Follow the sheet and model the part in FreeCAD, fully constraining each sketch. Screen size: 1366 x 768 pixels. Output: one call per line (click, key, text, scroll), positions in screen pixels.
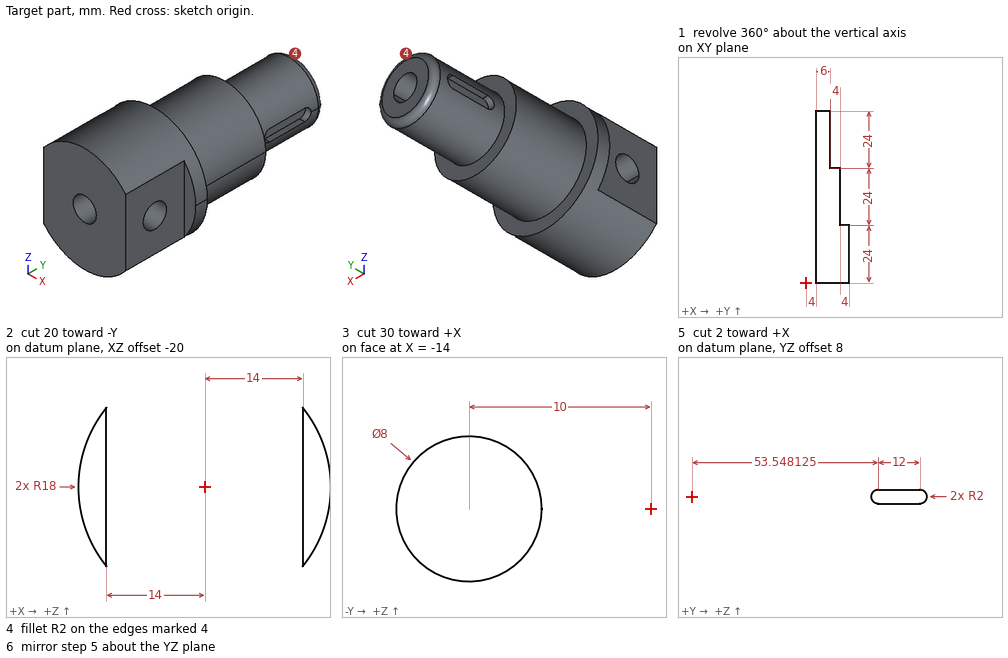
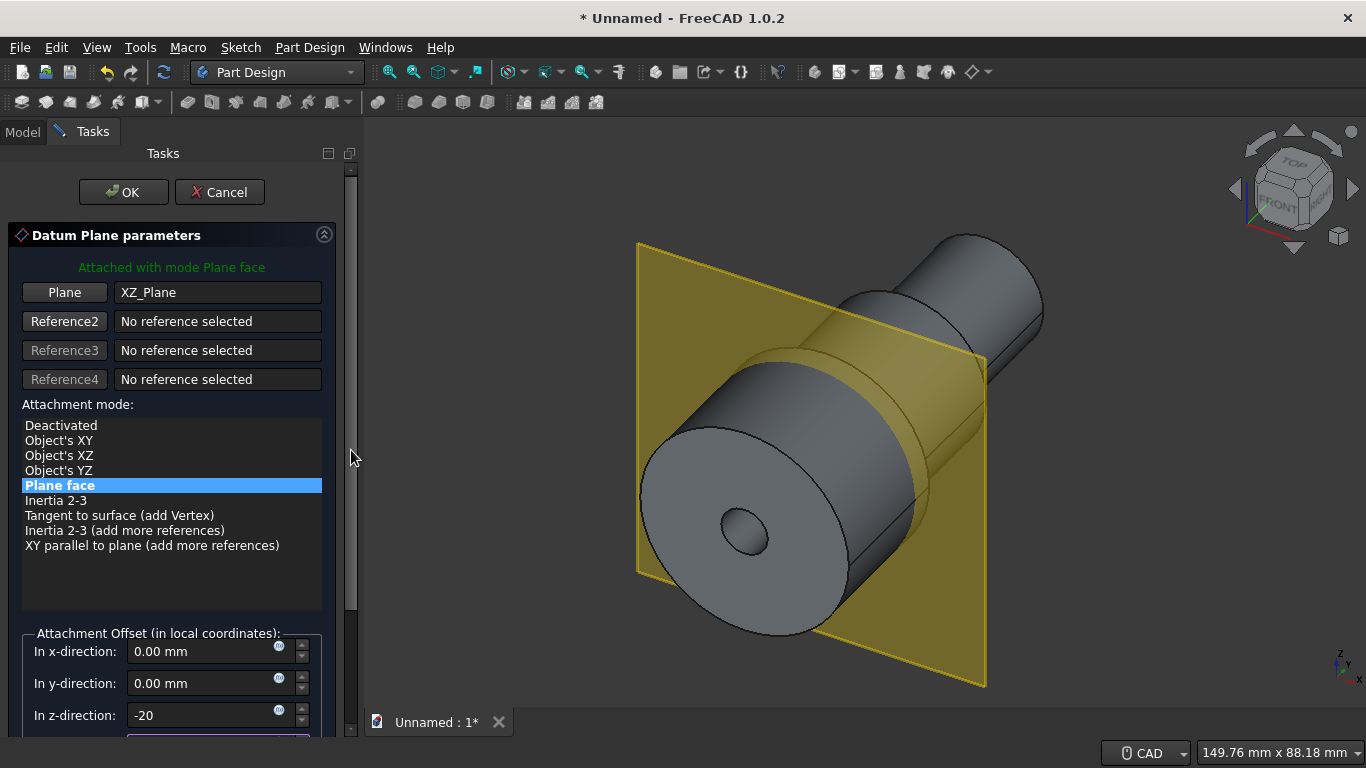
click(124, 192)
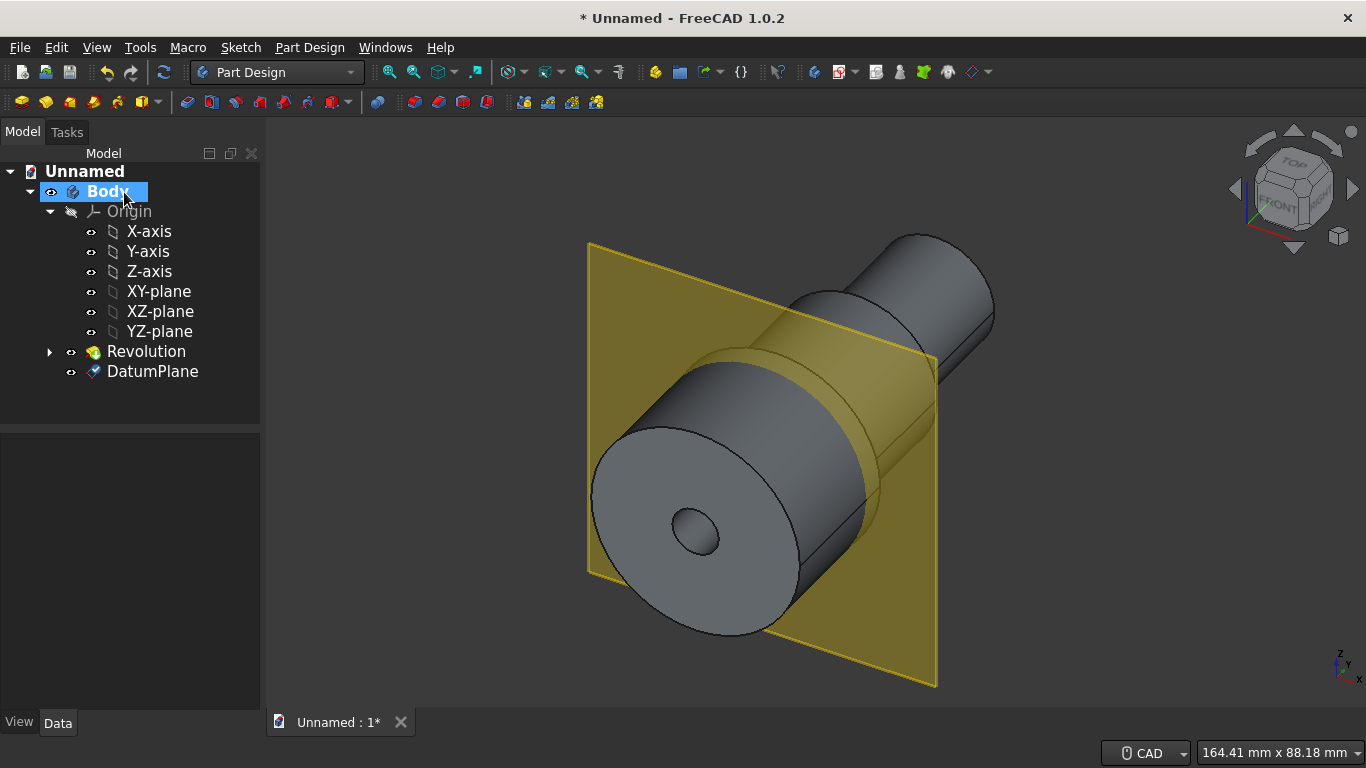
click(116, 372)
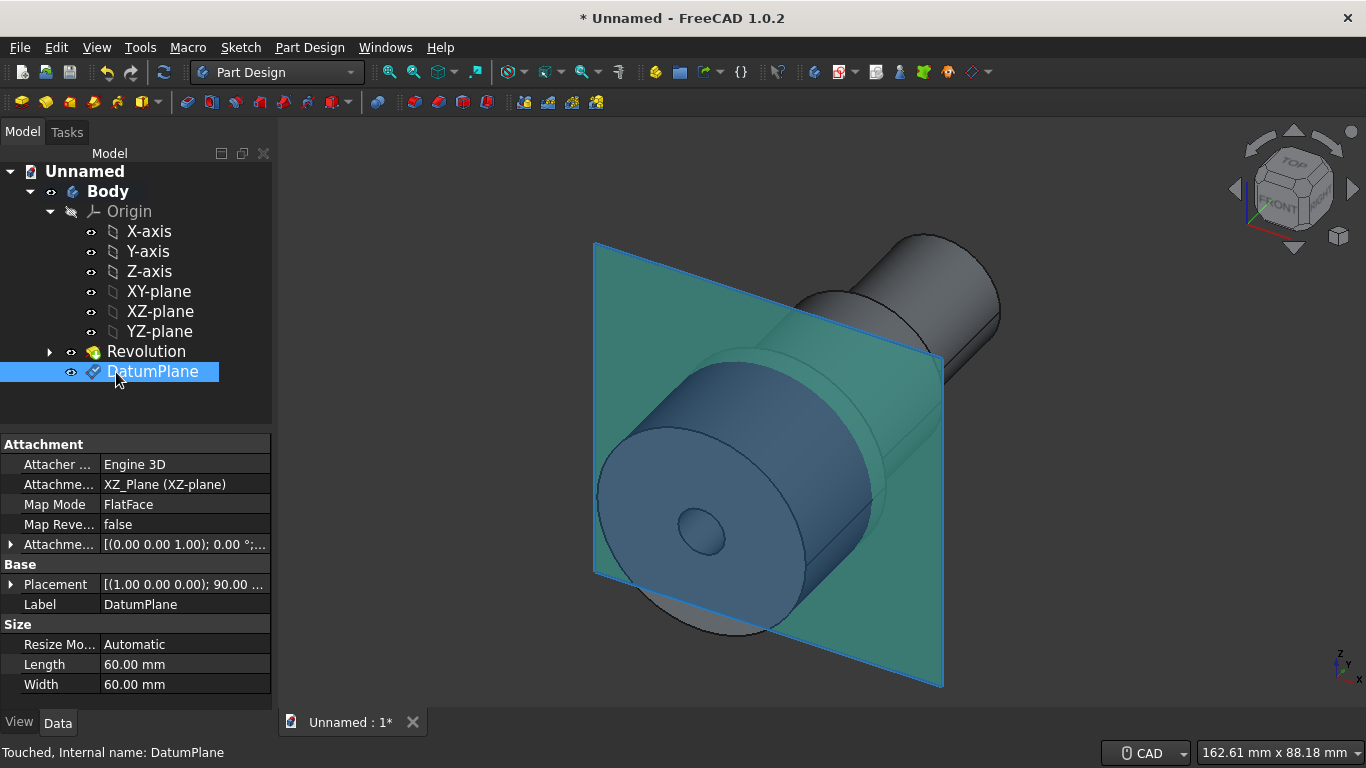
click(840, 72)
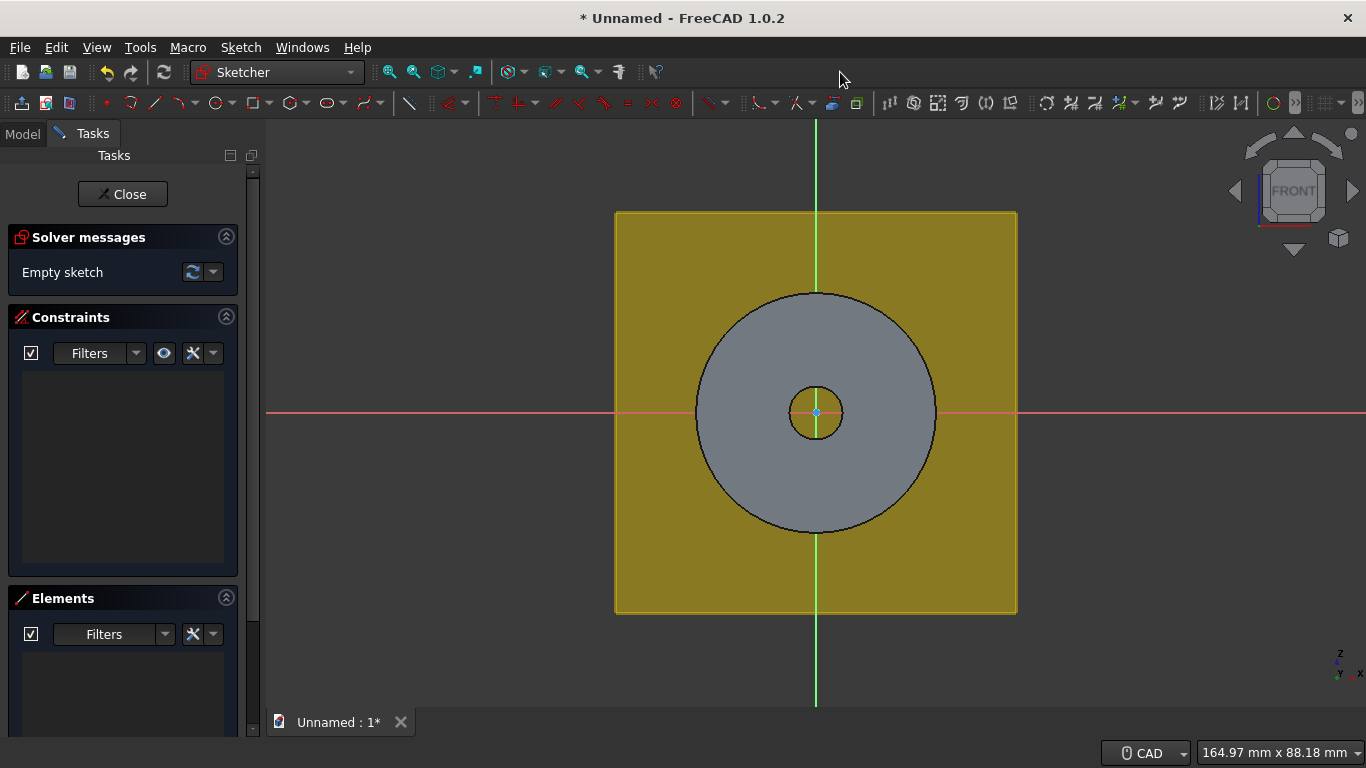
click(70, 104)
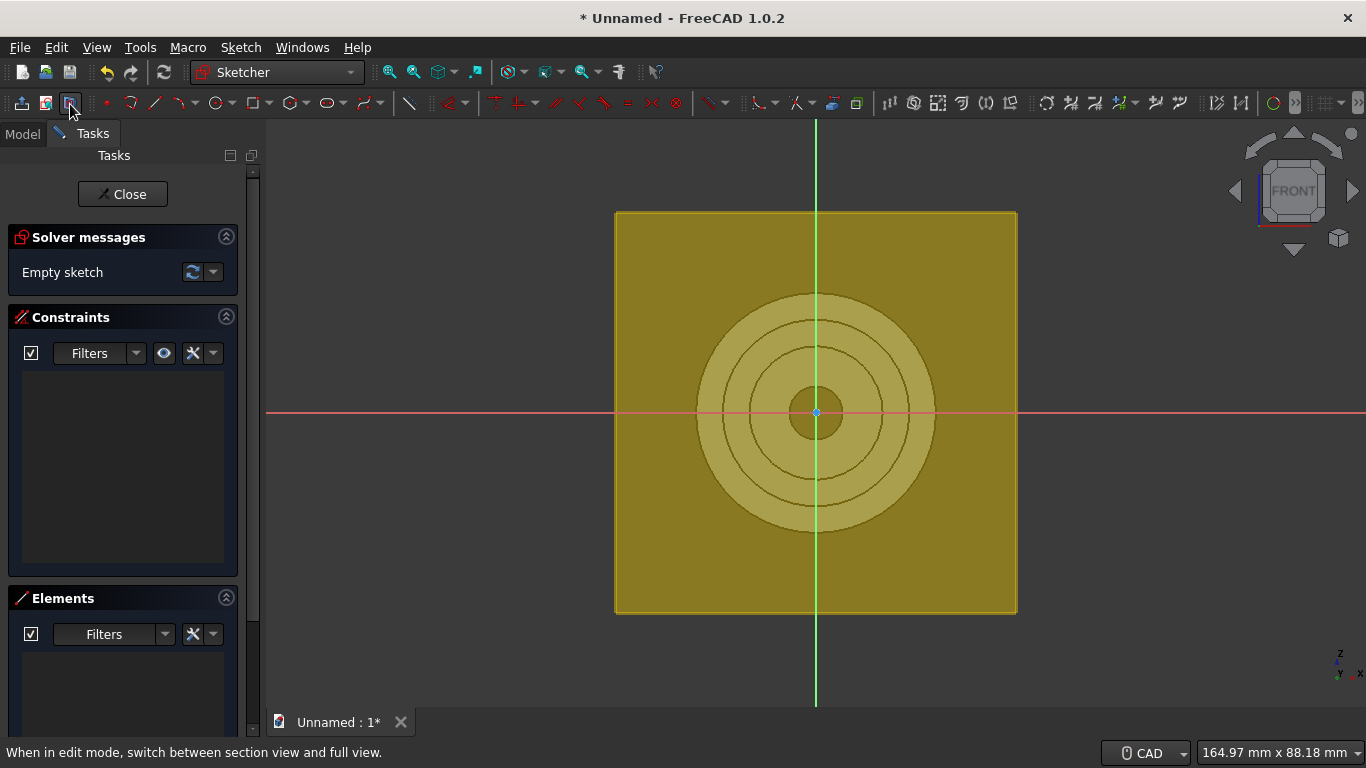
scroll(856, 413, up, 5)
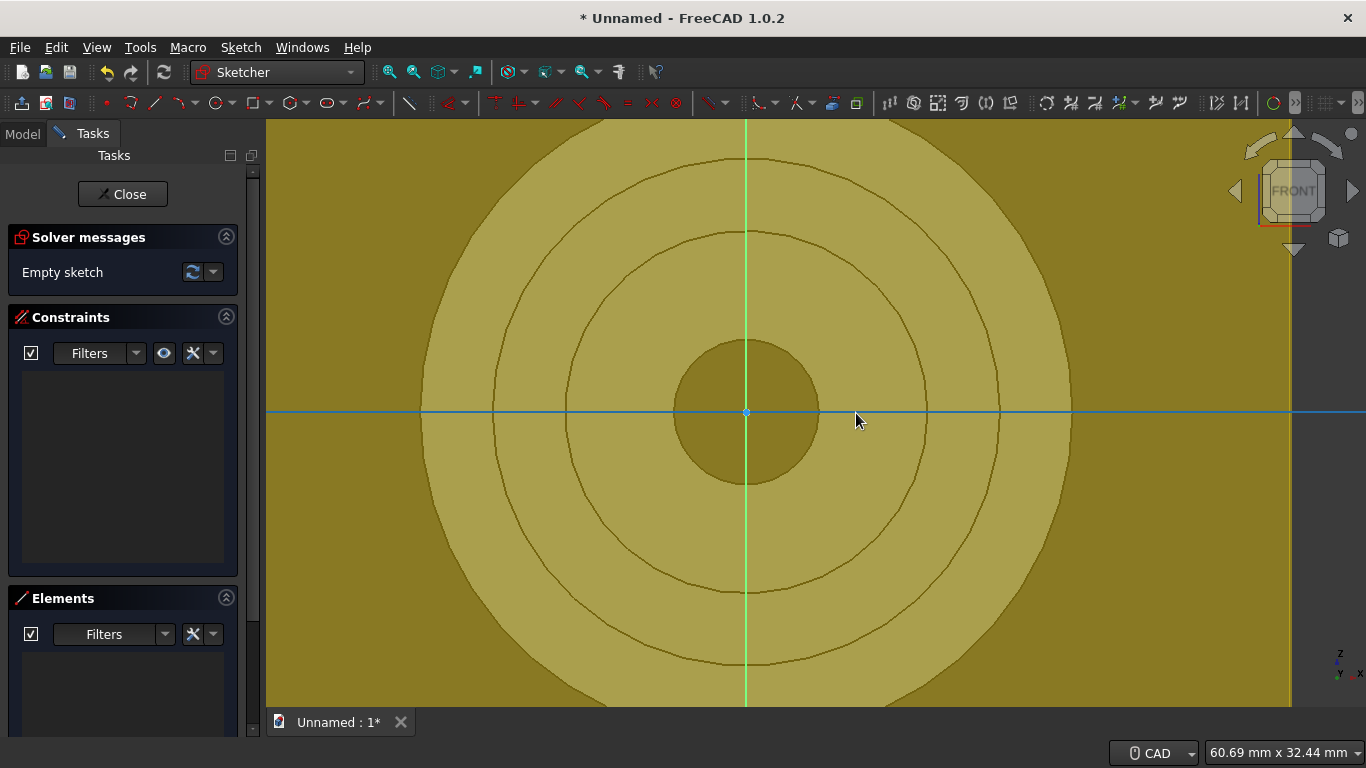
click(156, 104)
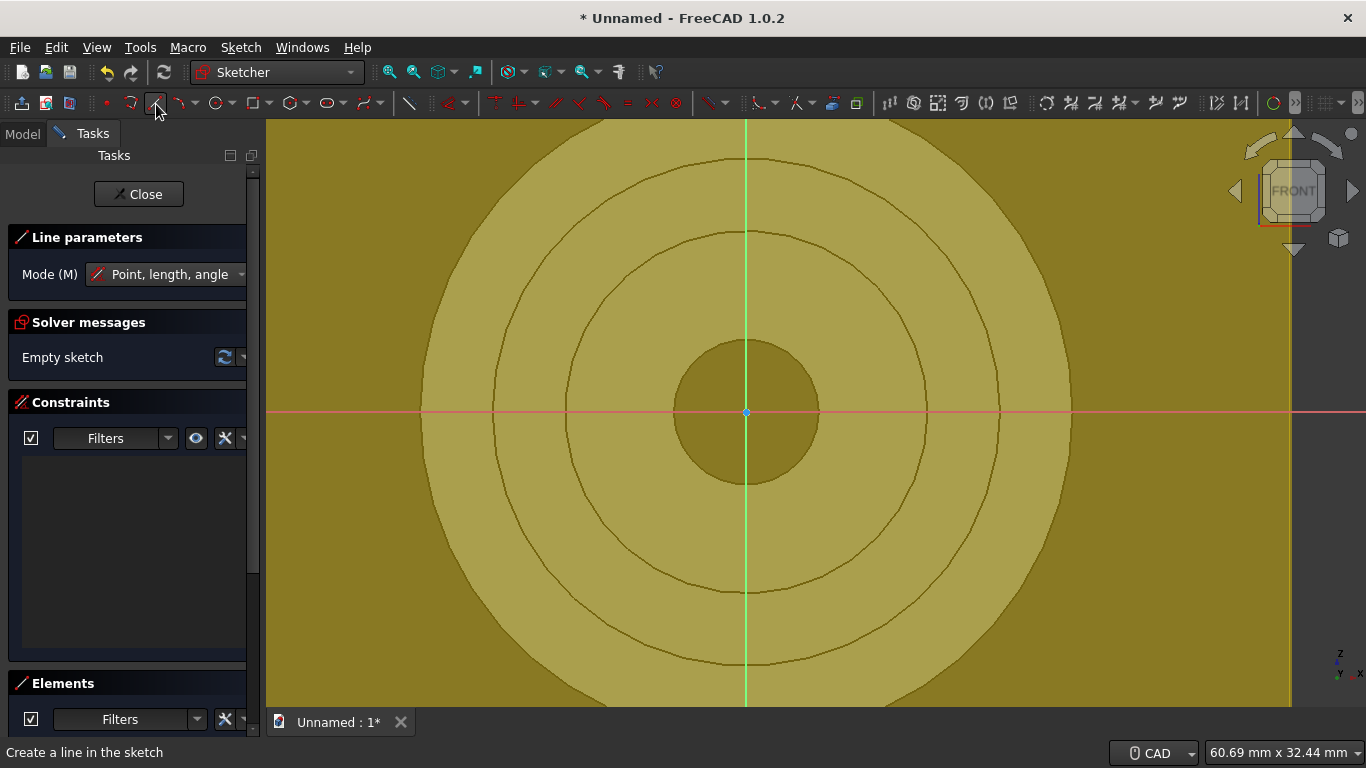
click(493, 617)
click(493, 207)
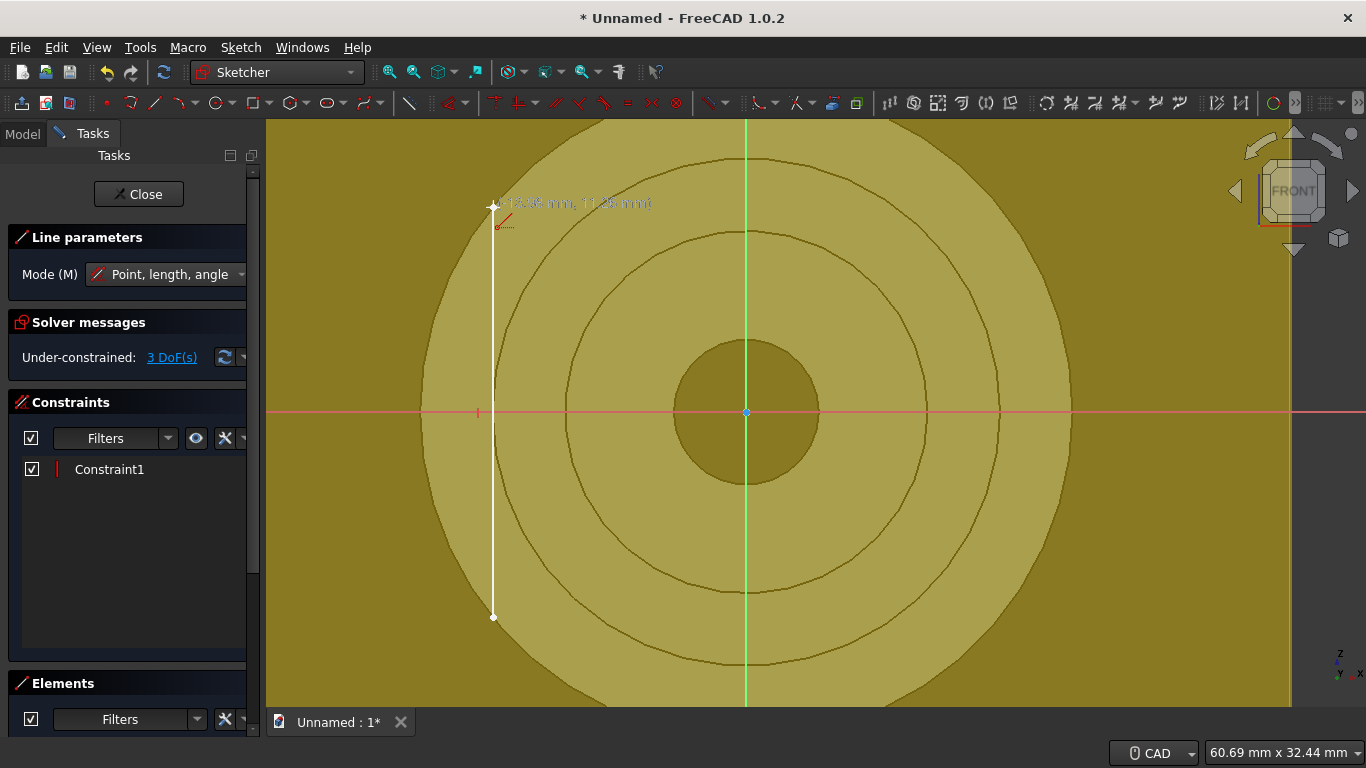
click(180, 104)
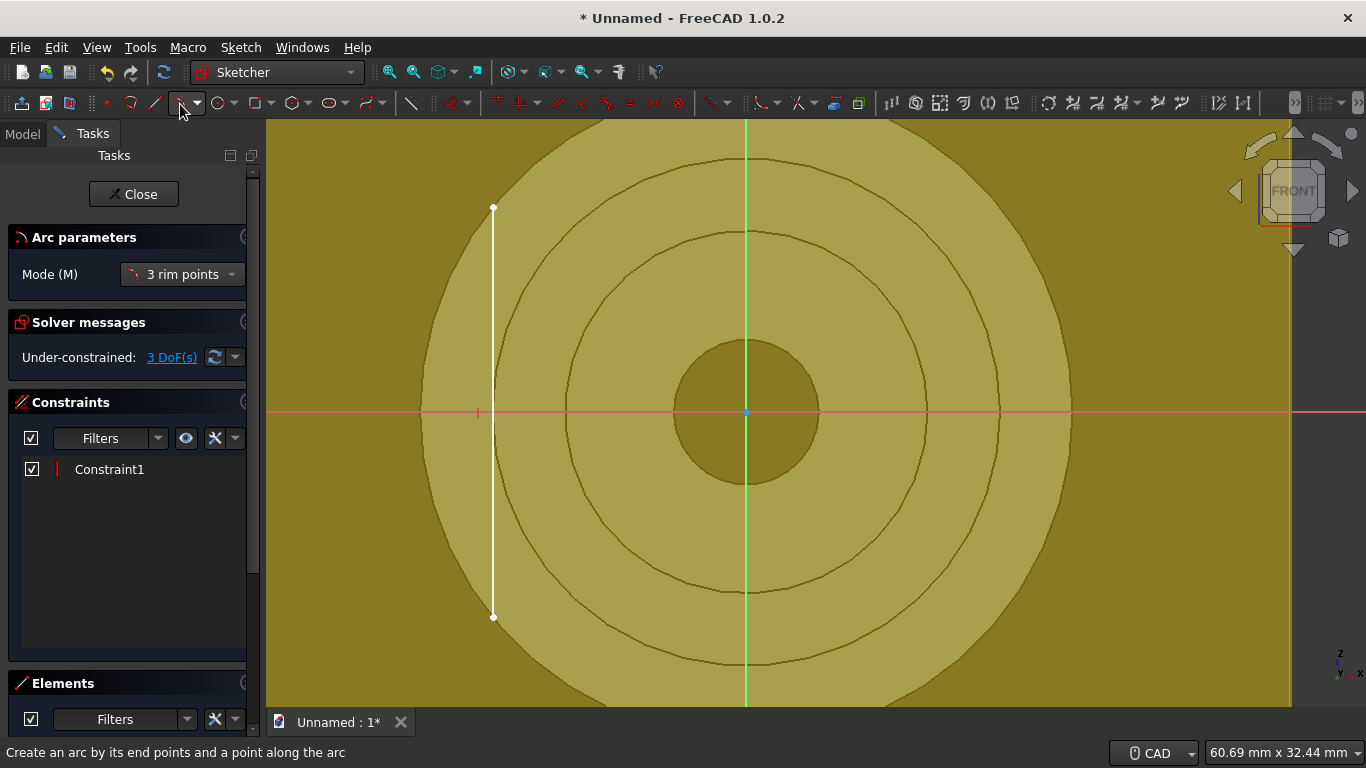
click(493, 208)
click(493, 618)
click(423, 368)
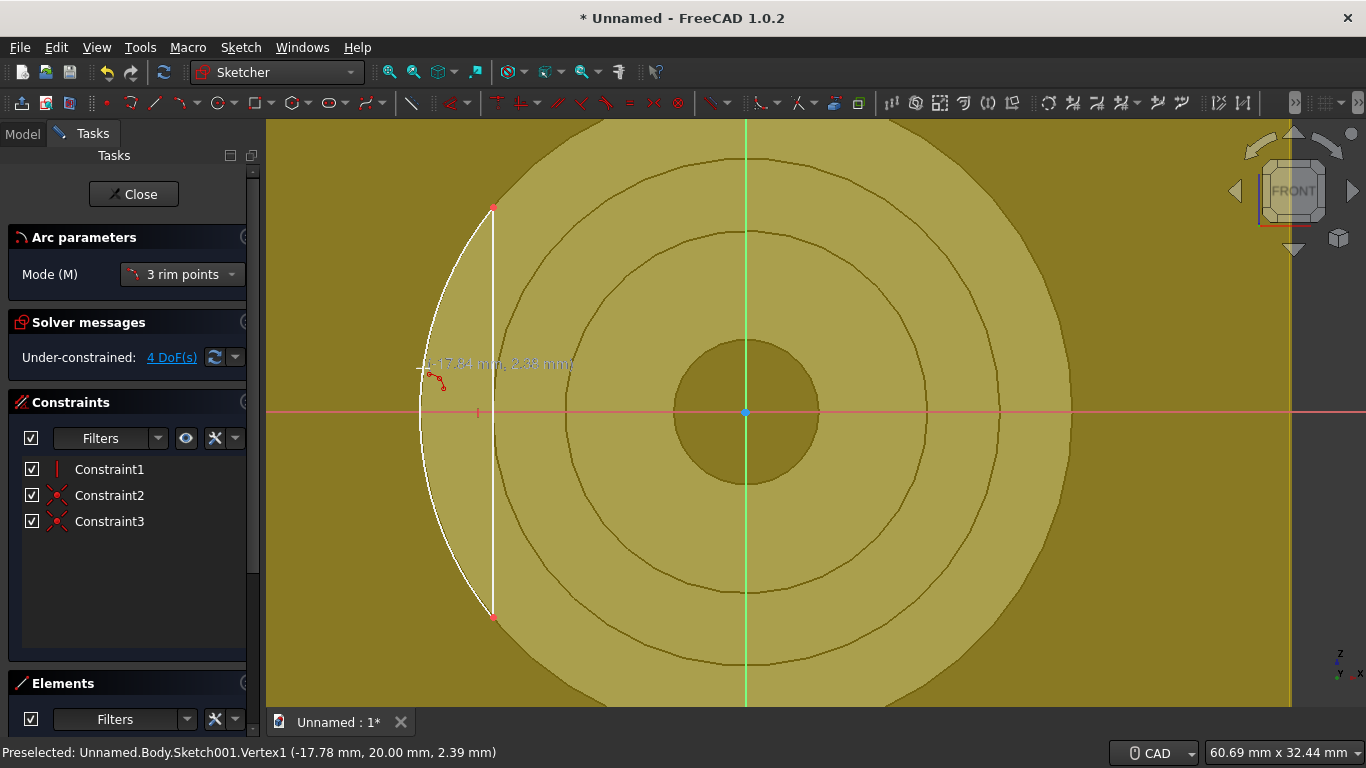
click(156, 104)